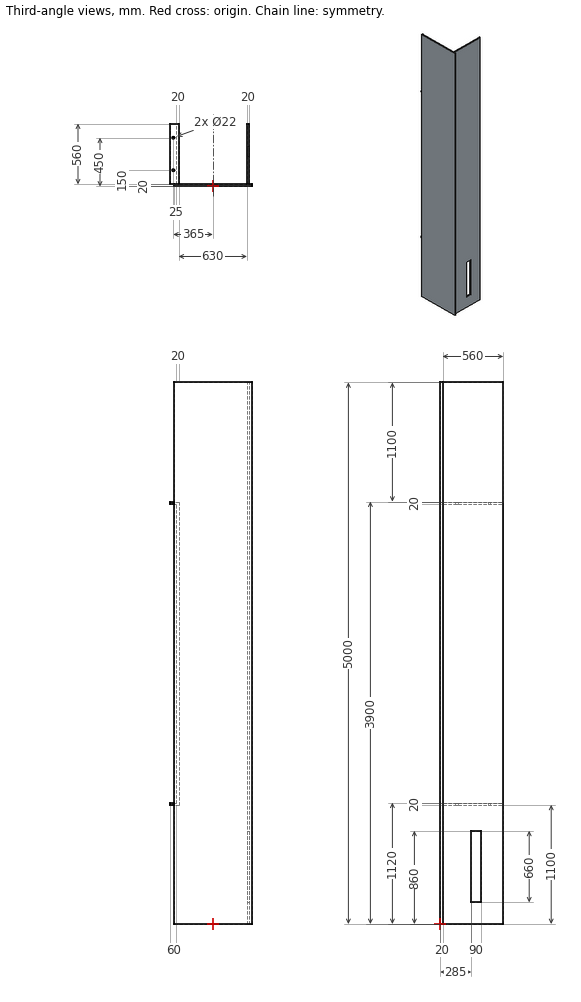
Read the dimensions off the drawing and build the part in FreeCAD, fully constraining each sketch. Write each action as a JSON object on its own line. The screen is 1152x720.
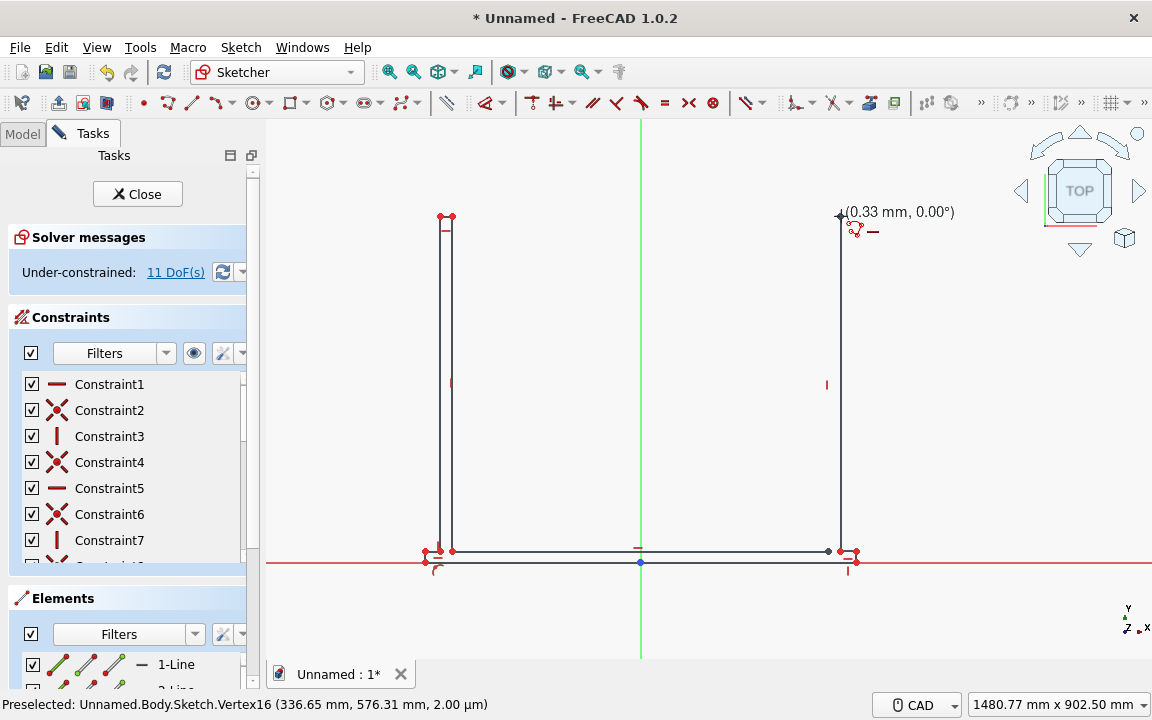
{"action": "scroll", "coordinate": [829, 216], "scroll_direction": "up", "scroll_amount": 2}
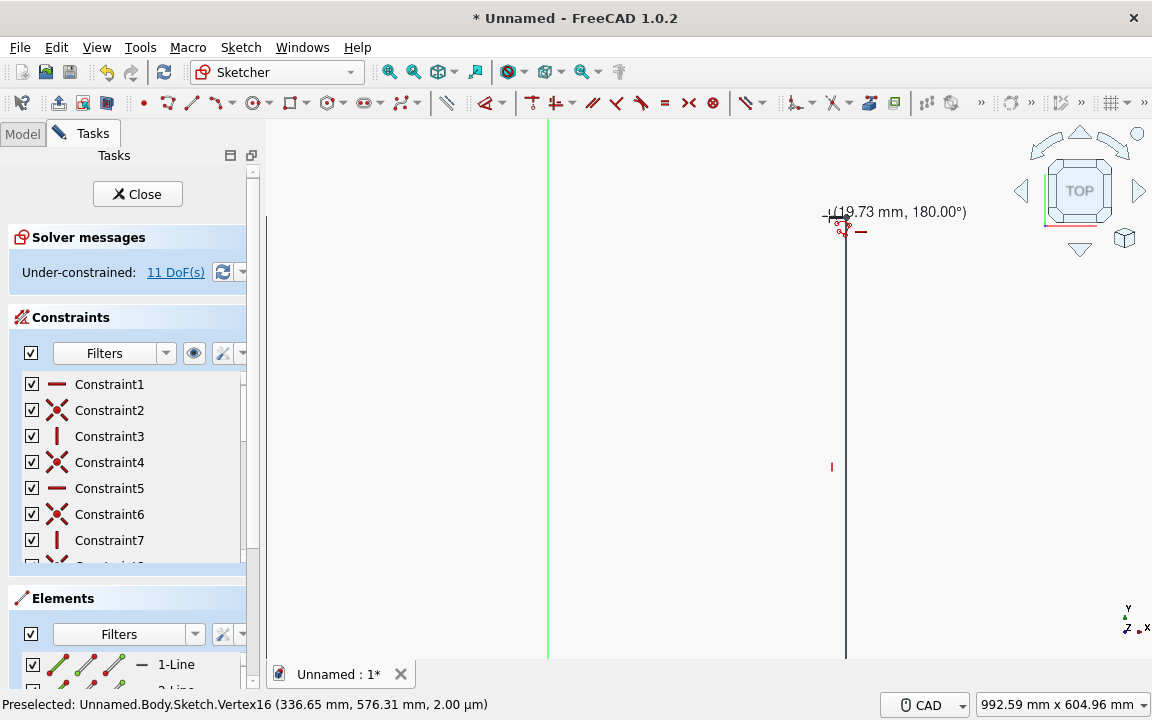
{"action": "left_click", "coordinate": [829, 216]}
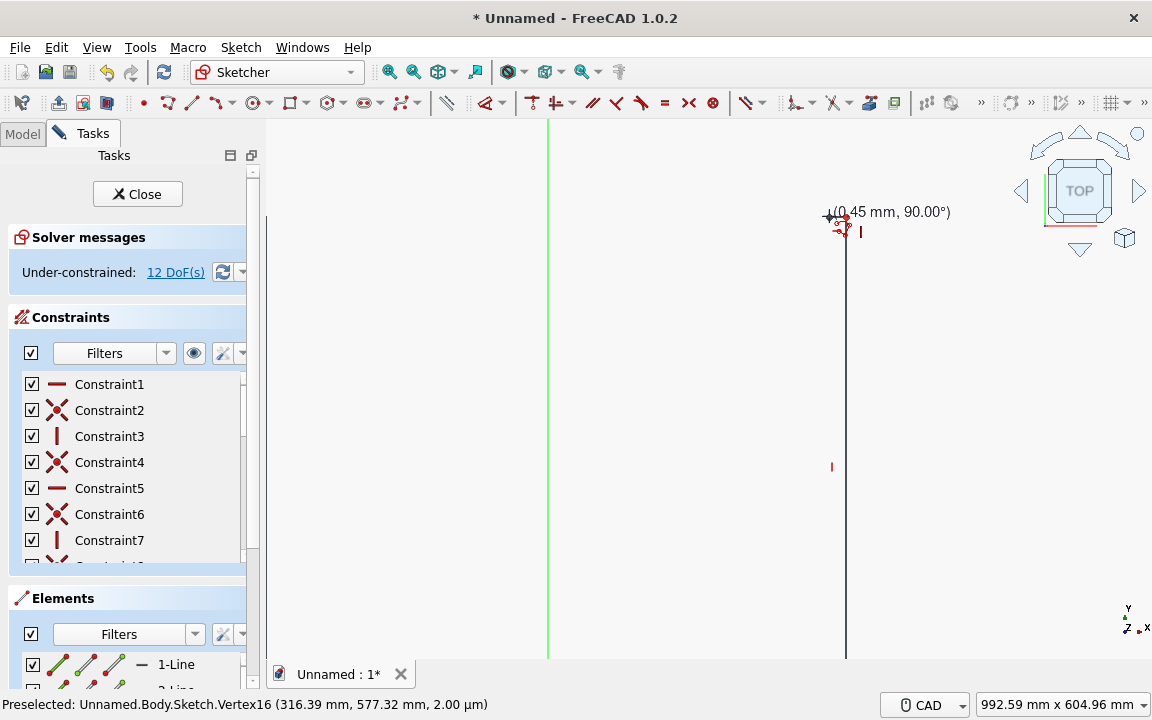
{"action": "scroll", "coordinate": [829, 215], "scroll_direction": "down", "scroll_amount": 2}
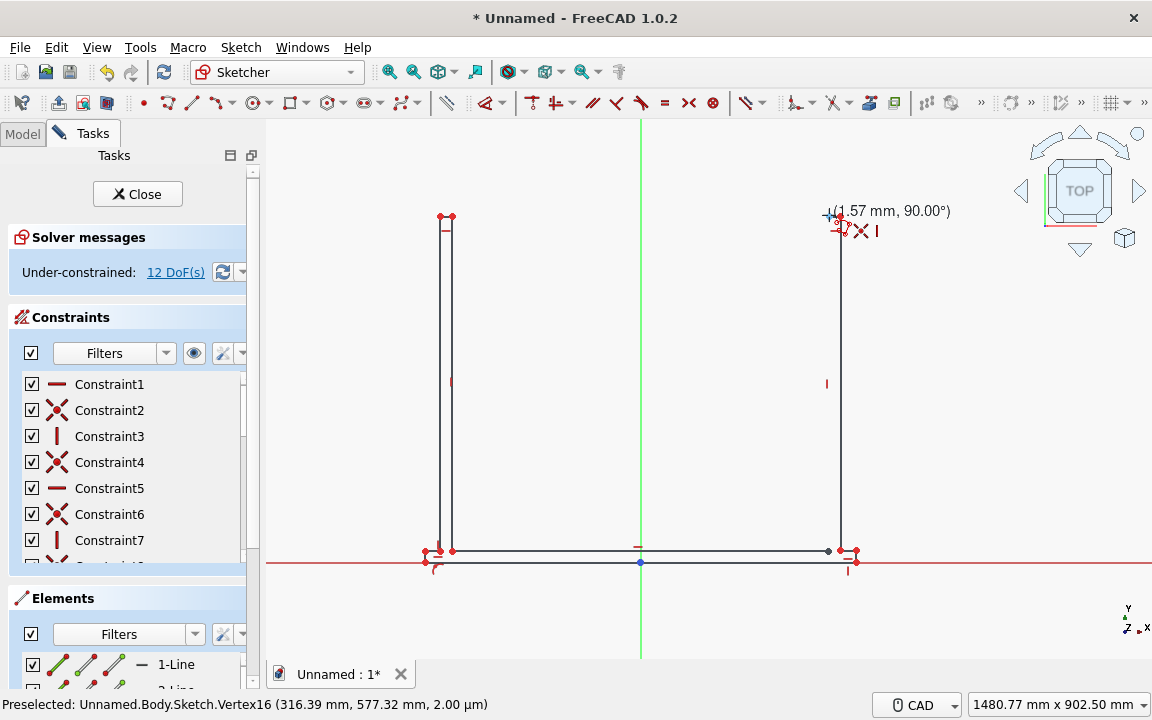
{"action": "scroll", "coordinate": [829, 551], "scroll_direction": "up", "scroll_amount": 2}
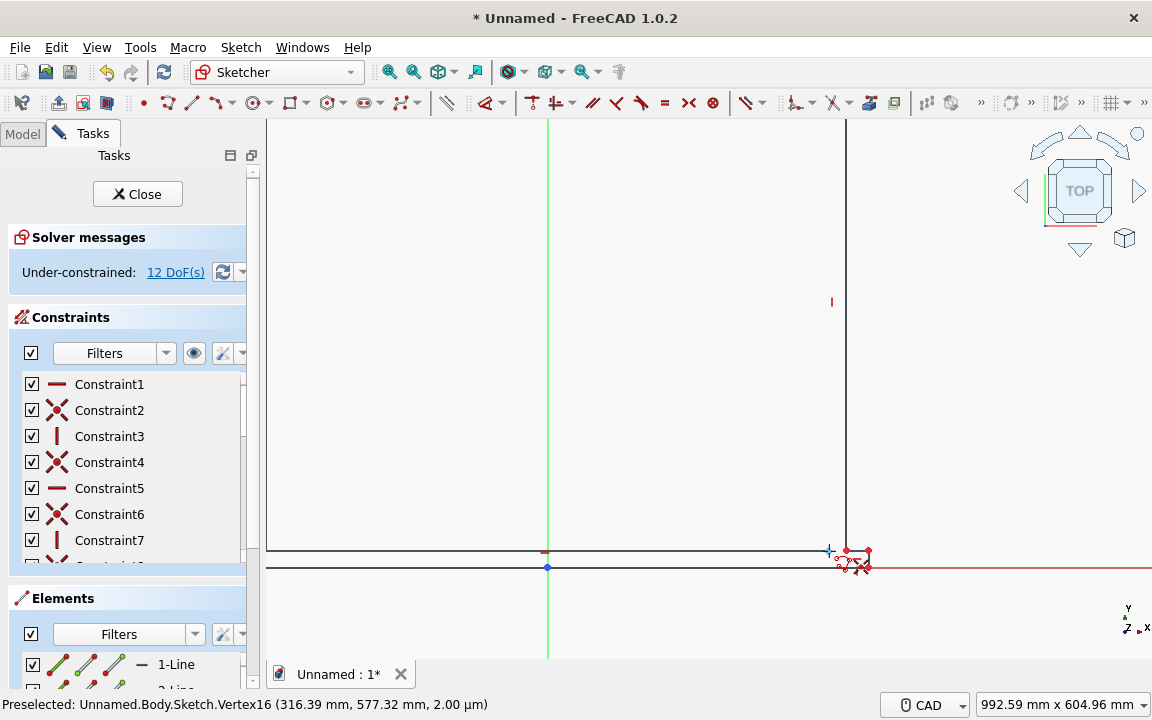
{"action": "left_click", "coordinate": [829, 551]}
{"action": "key", "text": "Escape"}
{"action": "key", "text": "Escape"}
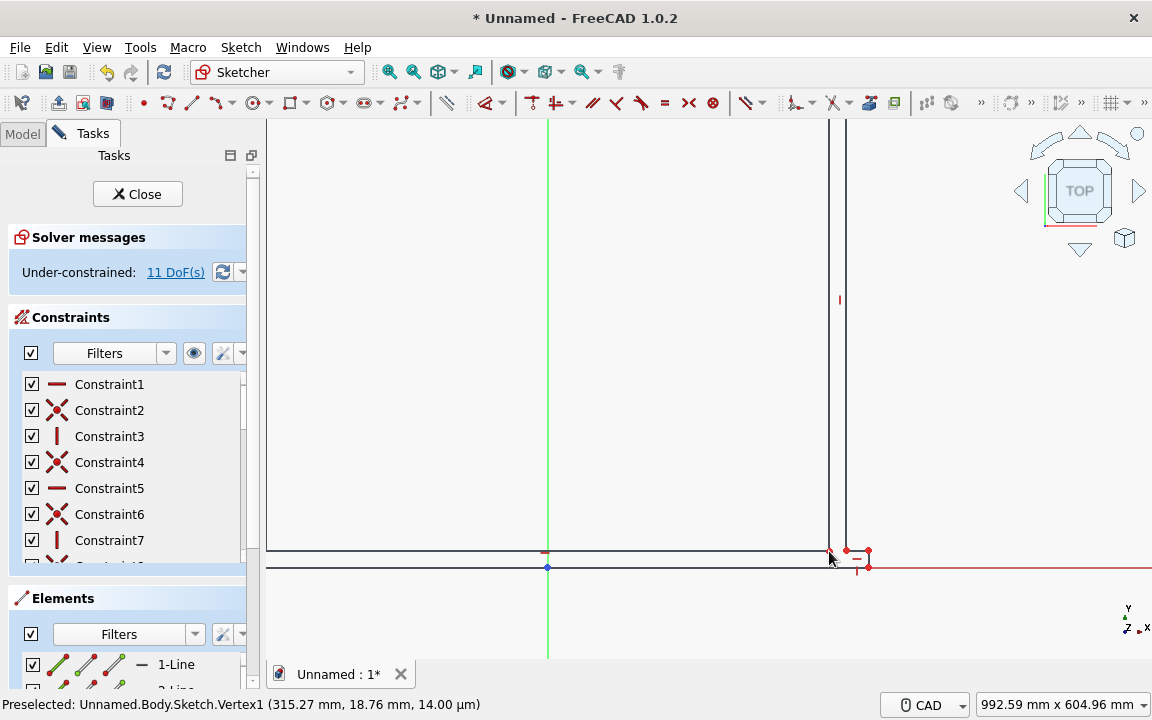
{"action": "scroll", "coordinate": [829, 552], "scroll_direction": "down", "scroll_amount": 2}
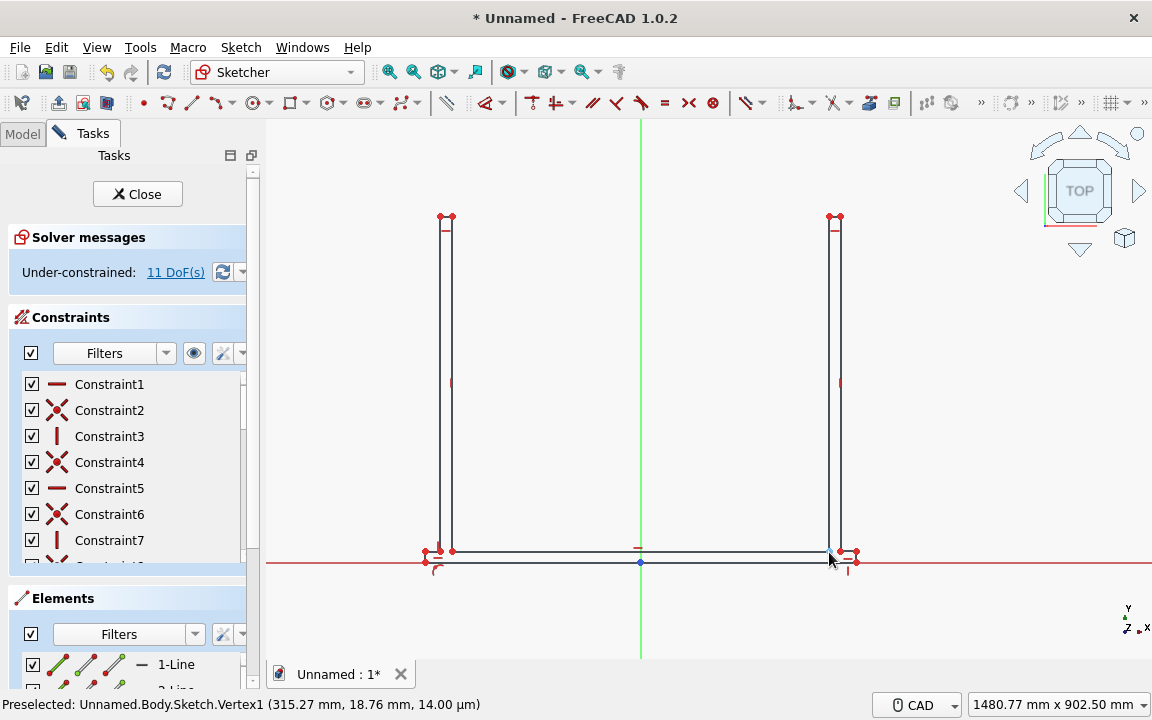
{"action": "left_click", "coordinate": [425, 552]}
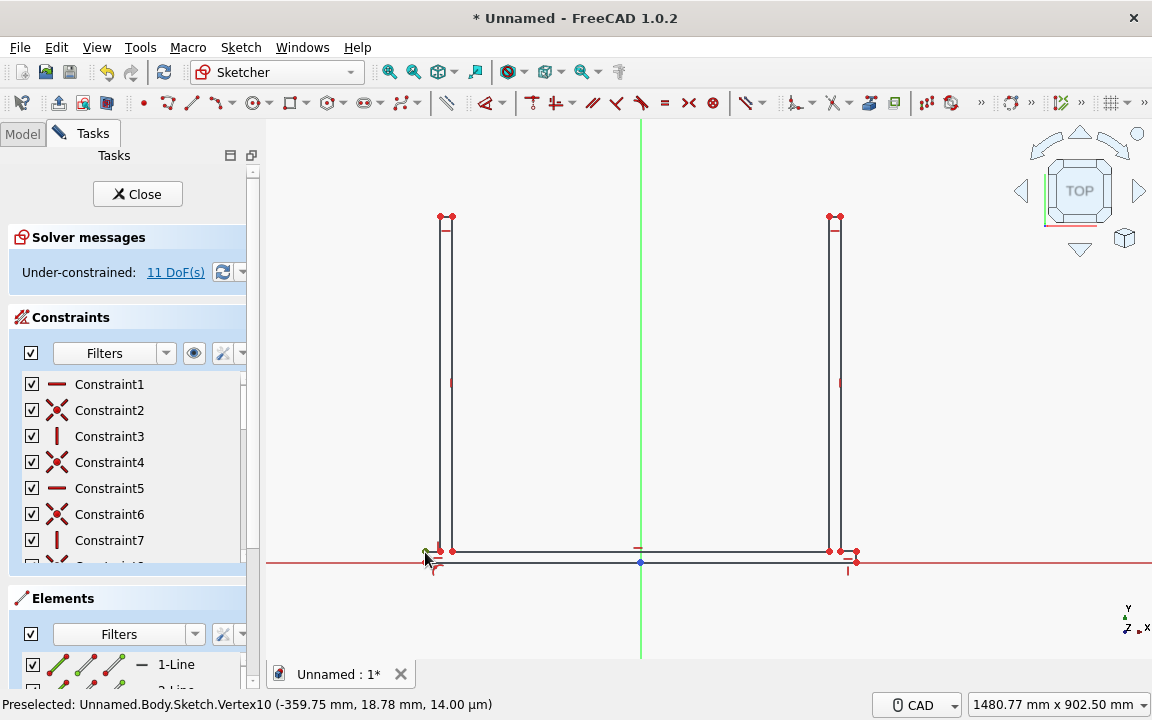
{"action": "left_click", "coordinate": [856, 551]}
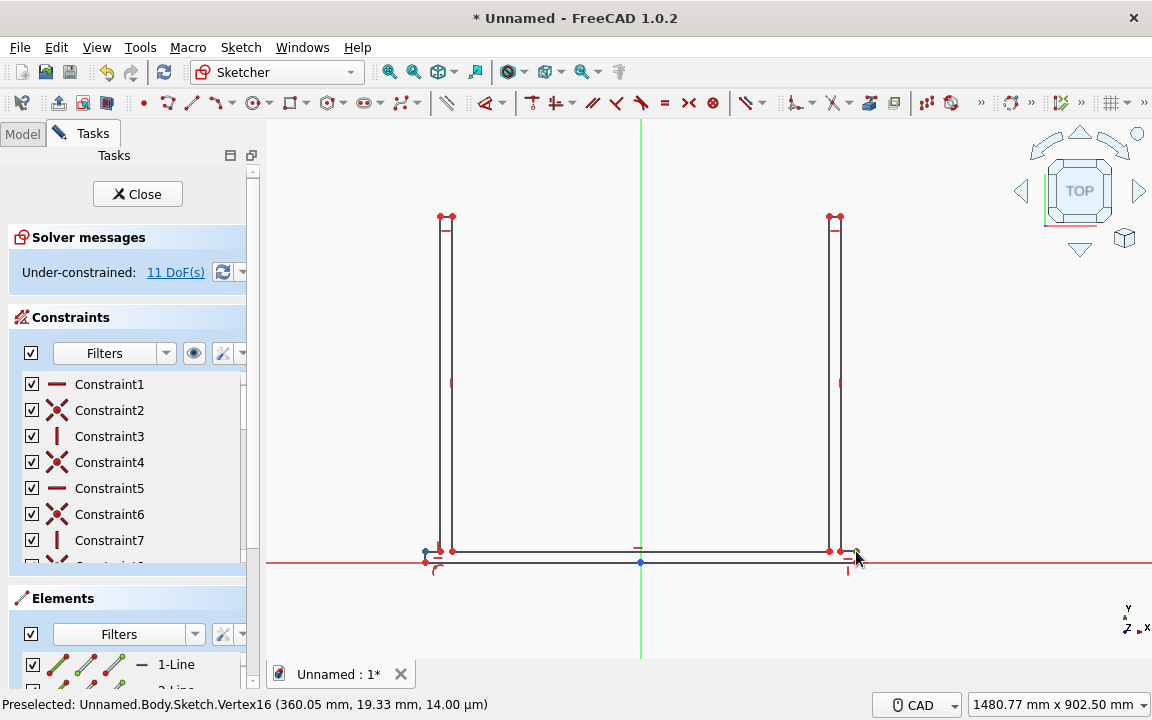
{"action": "left_click", "coordinate": [641, 596]}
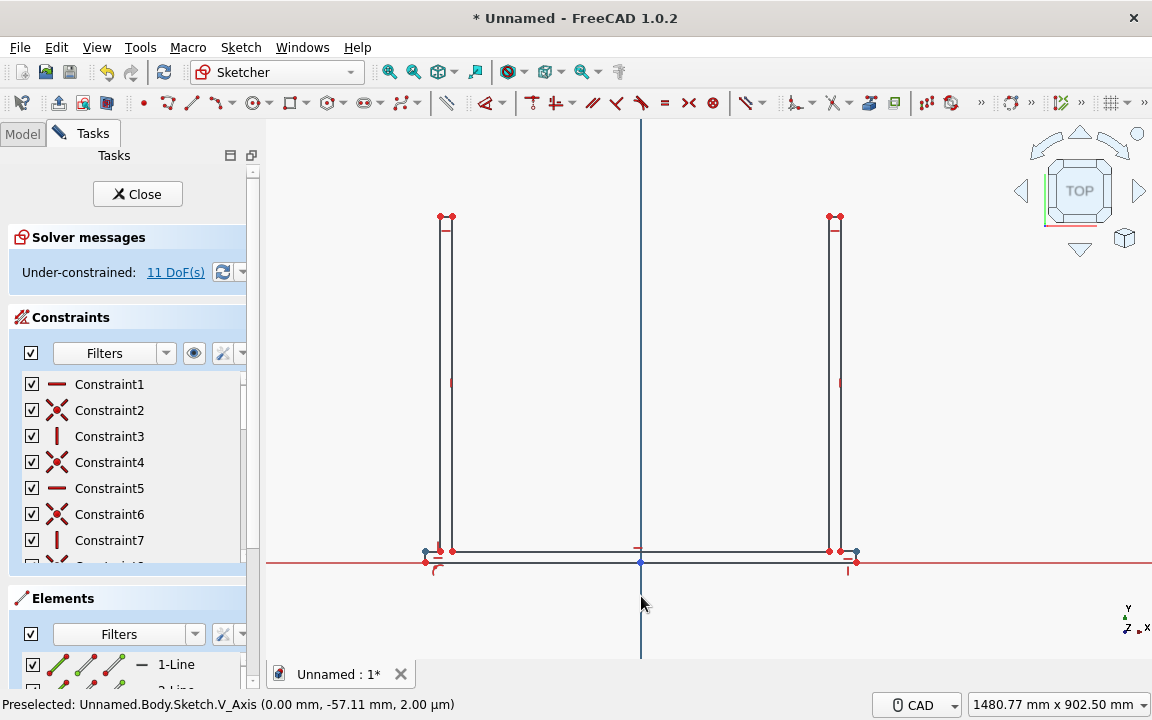
{"action": "left_click", "coordinate": [690, 104]}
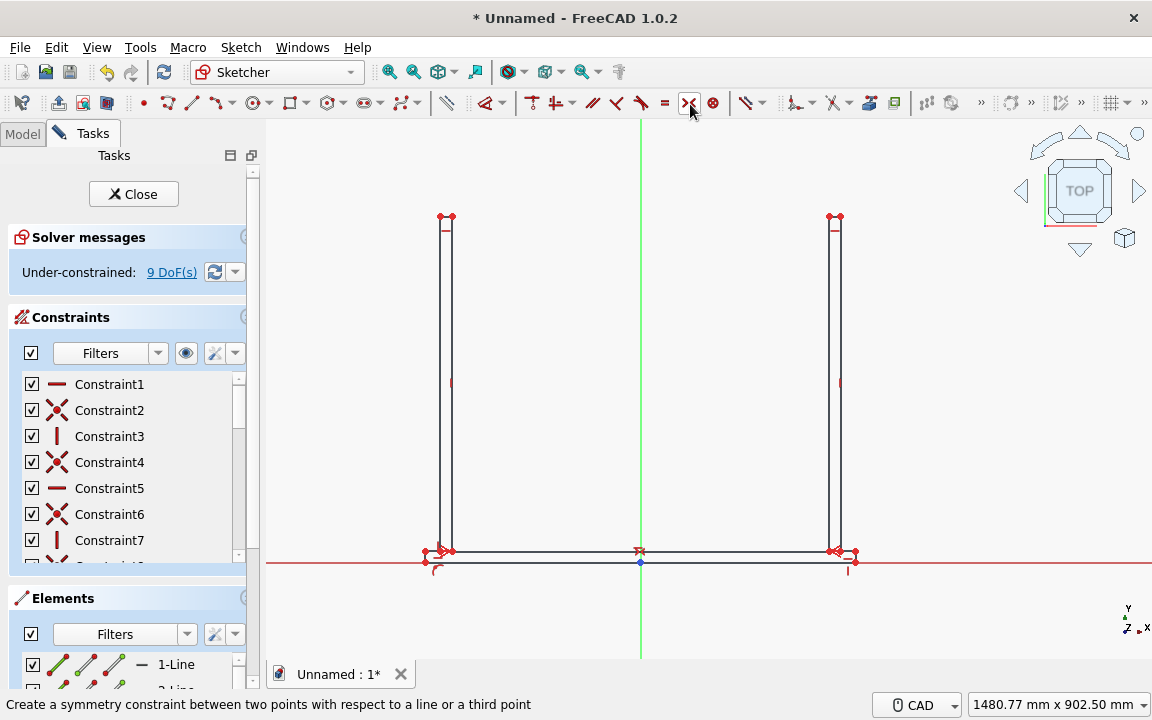
{"action": "left_click", "coordinate": [440, 217]}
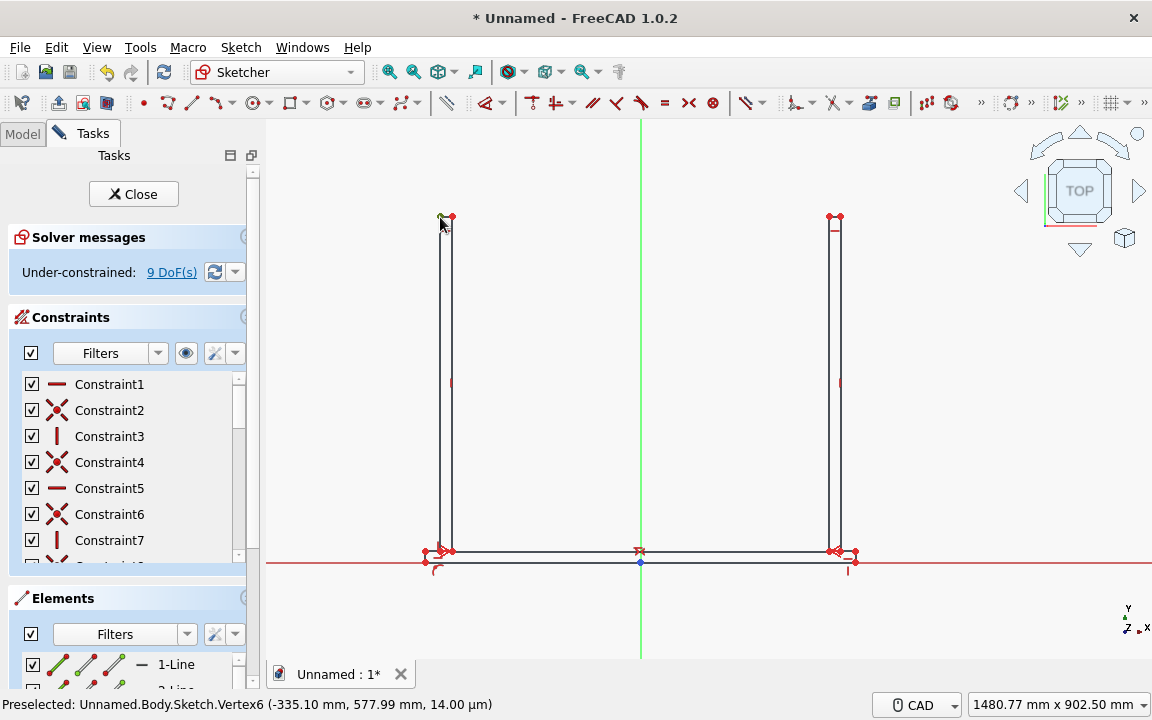
{"action": "left_click", "coordinate": [841, 217]}